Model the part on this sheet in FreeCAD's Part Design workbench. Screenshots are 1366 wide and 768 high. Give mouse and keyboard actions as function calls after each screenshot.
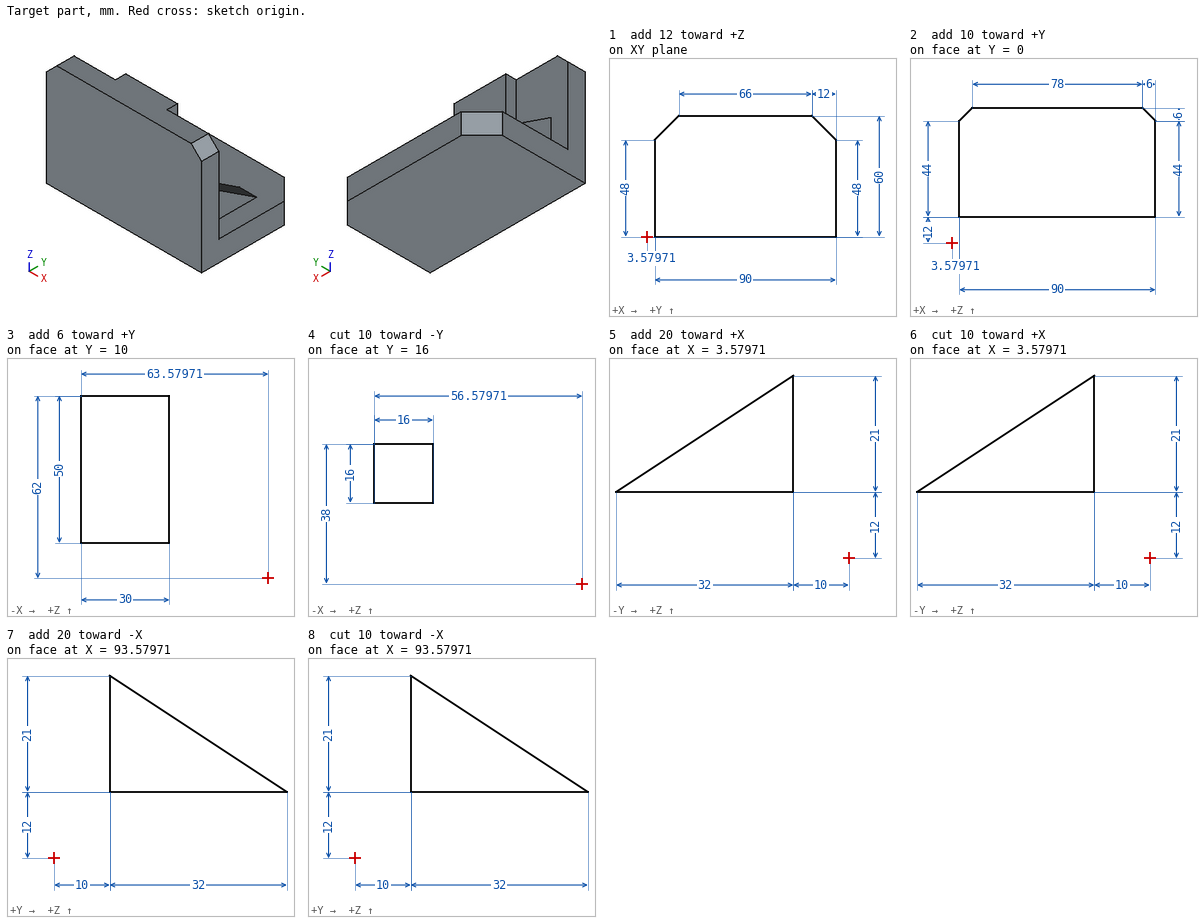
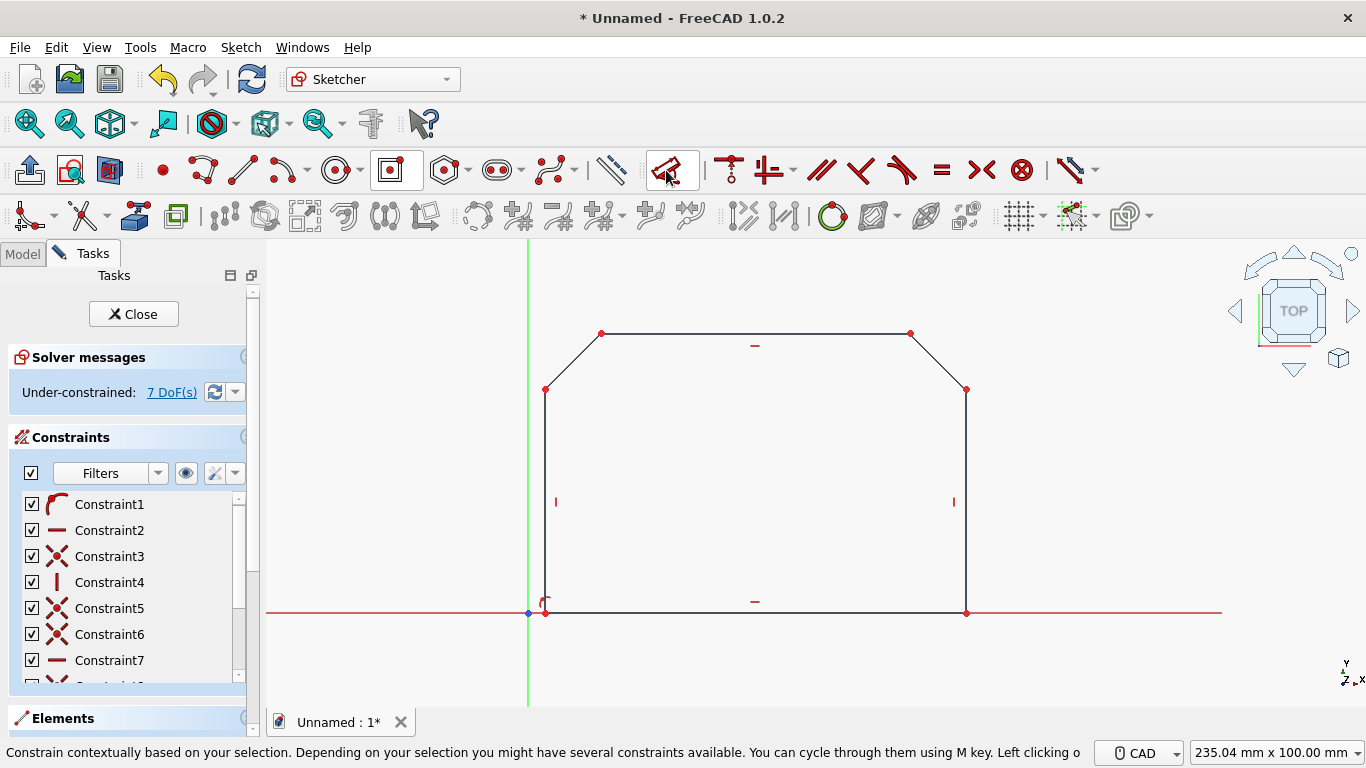
click(671, 613)
click(755, 647)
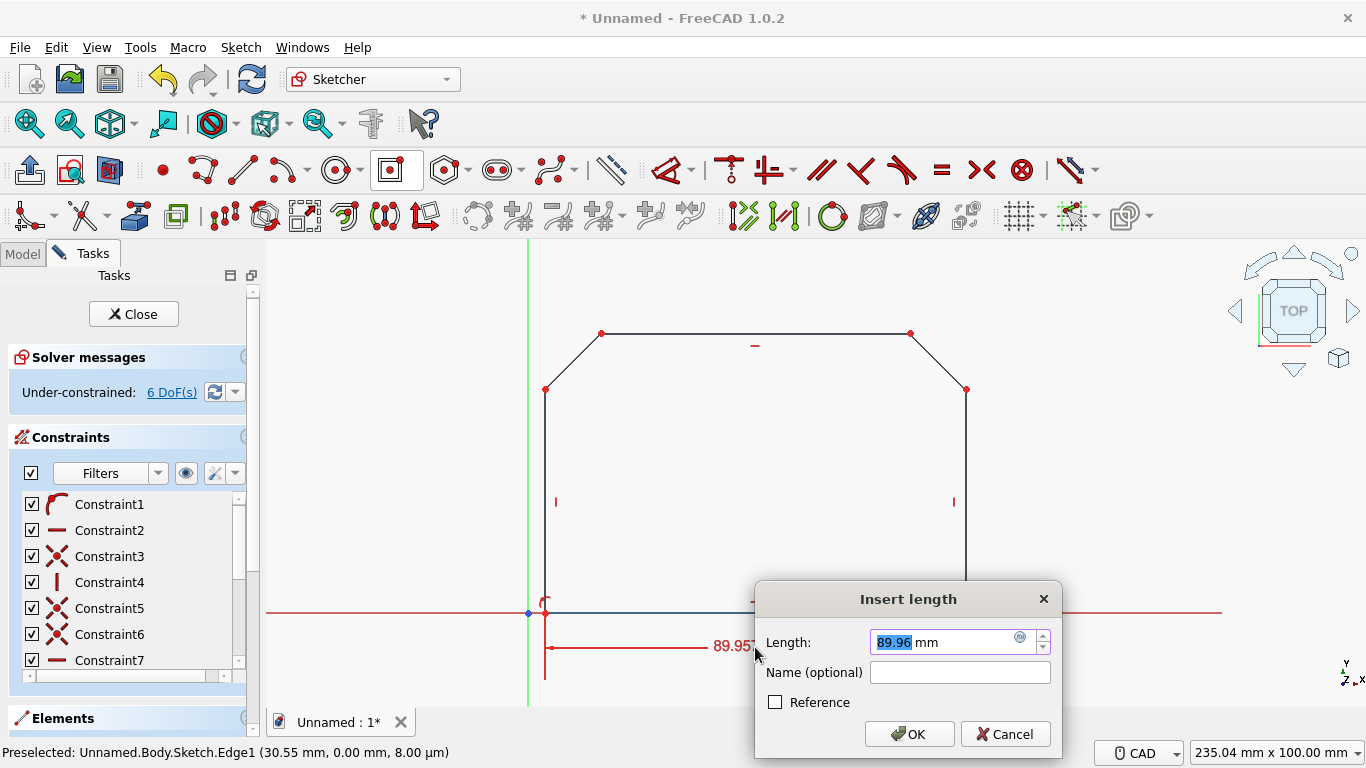
text(90)
key(Return)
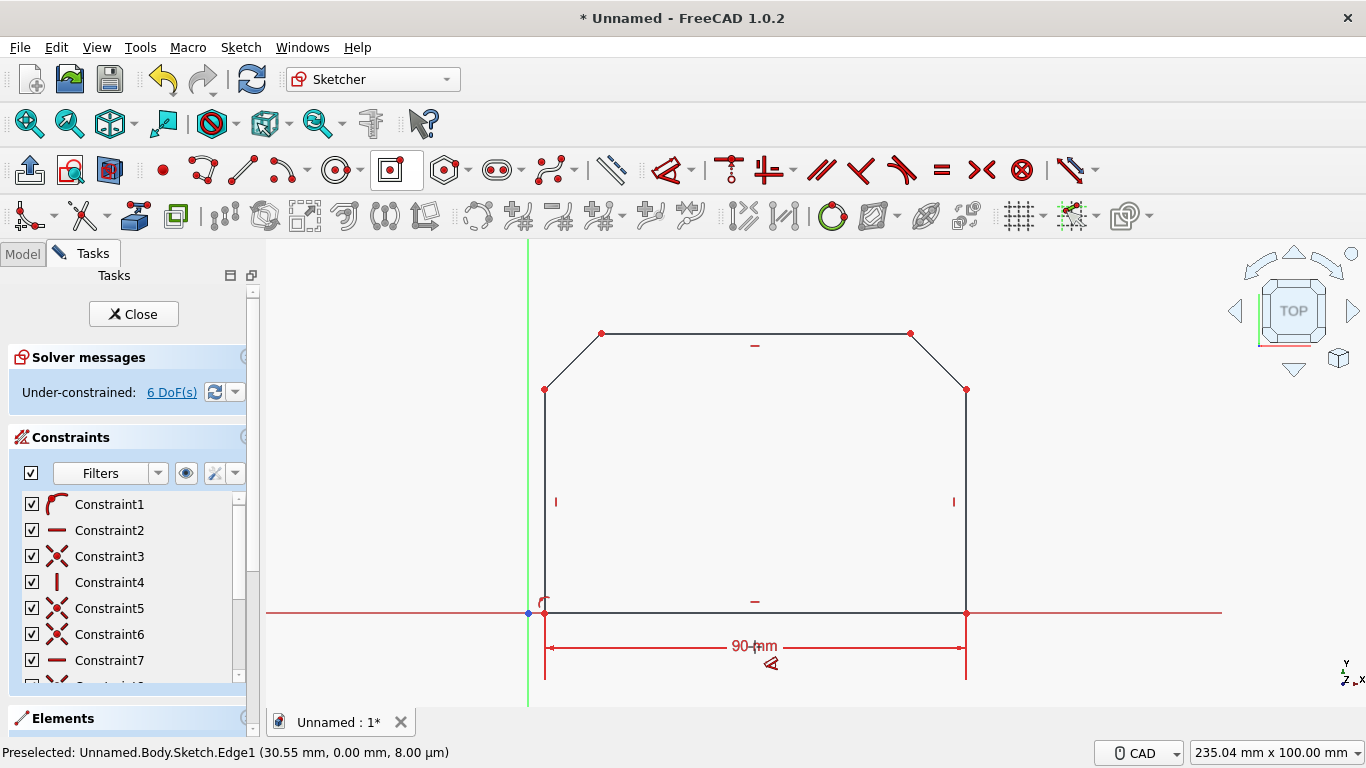
click(966, 546)
click(1000, 502)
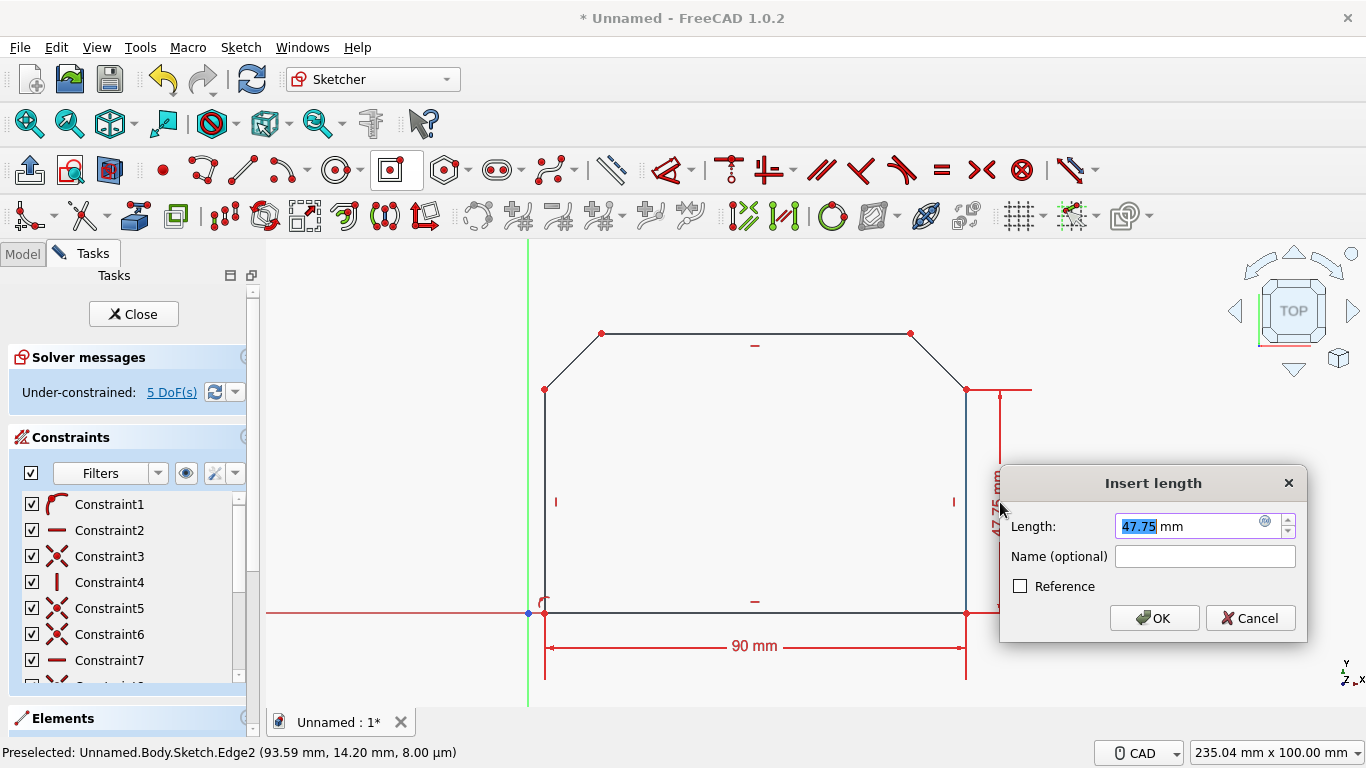
text(48)
key(Return)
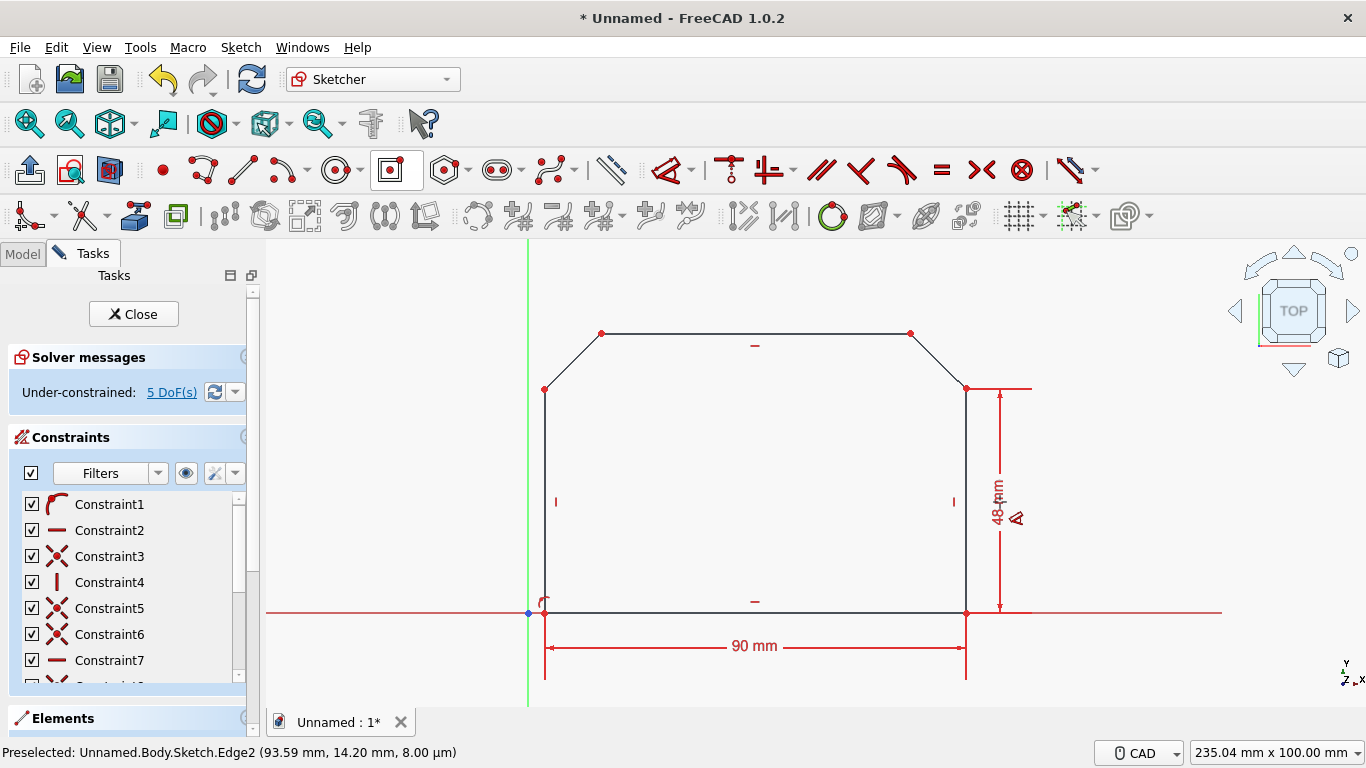
click(817, 334)
click(755, 300)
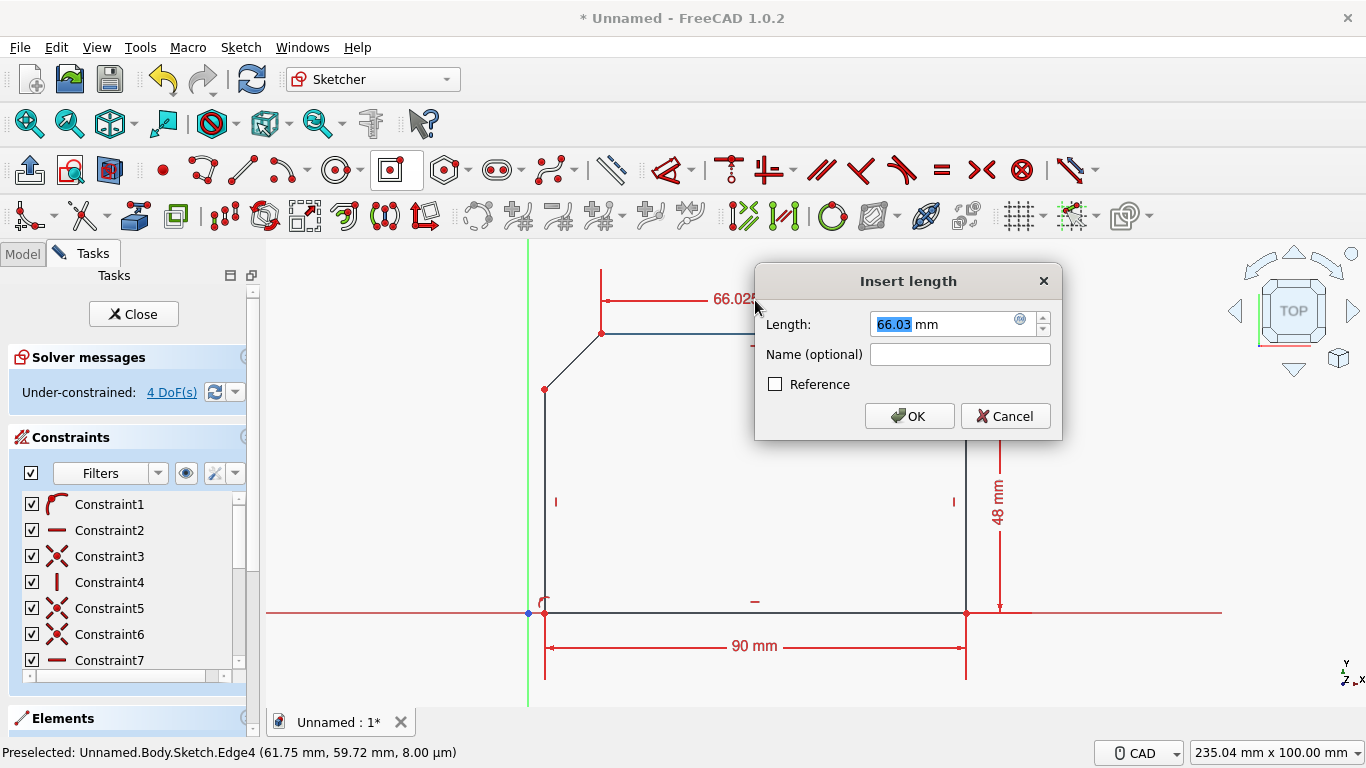
text(66)
key(Return)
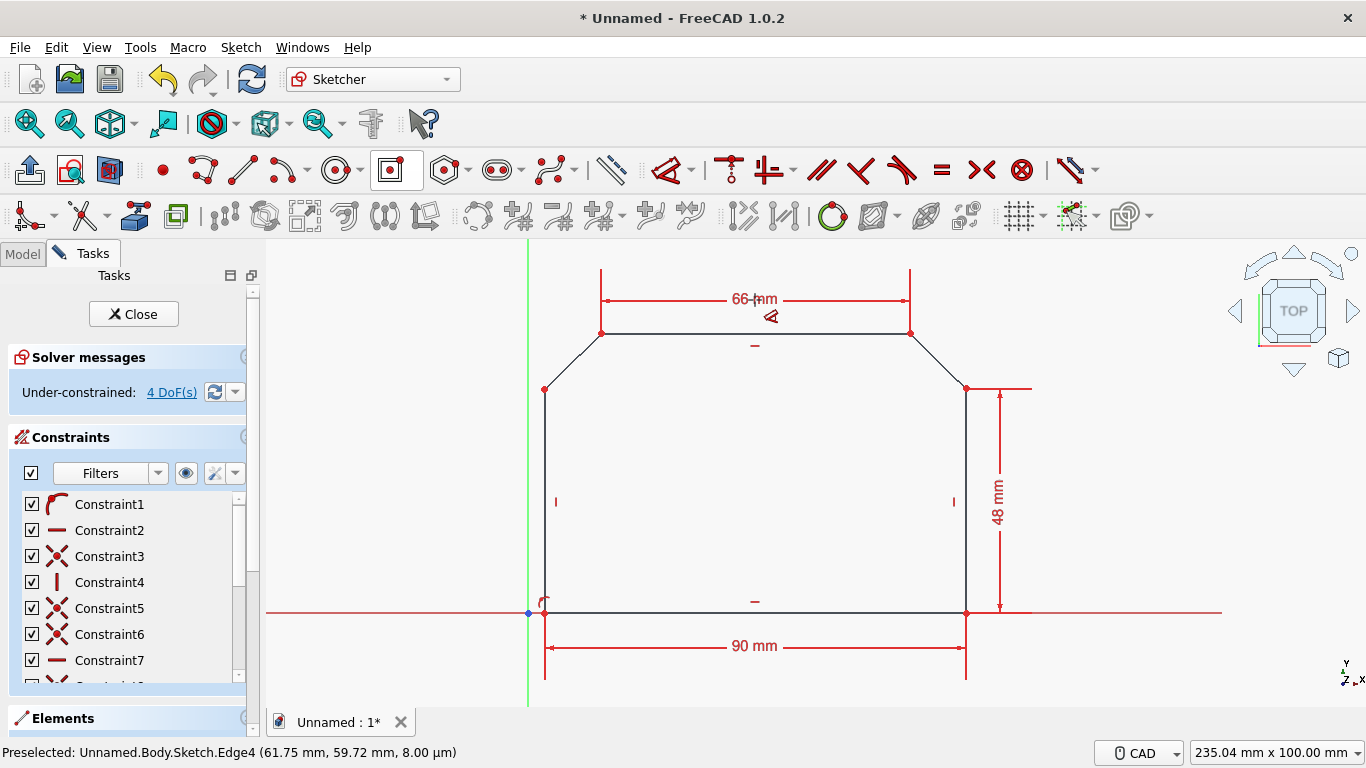
click(545, 457)
click(511, 502)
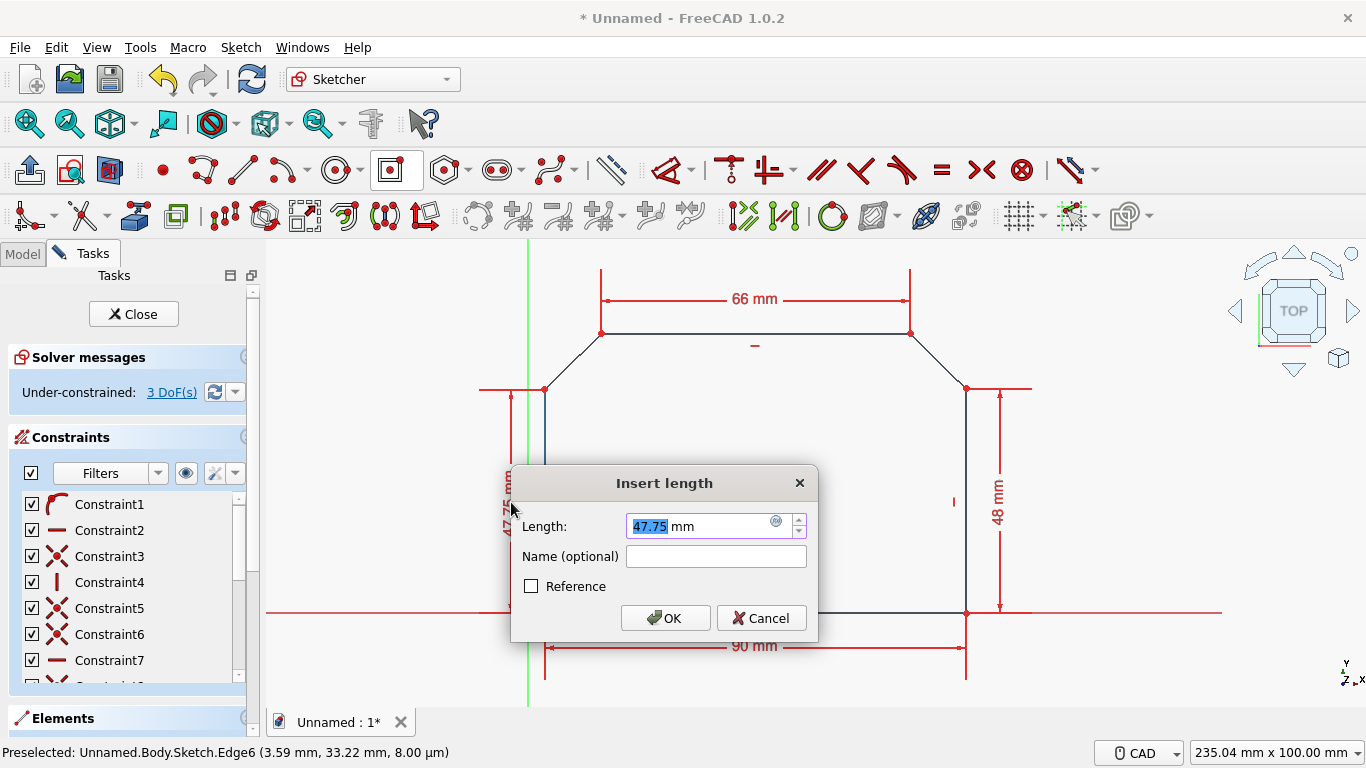
text(48)
key(Return)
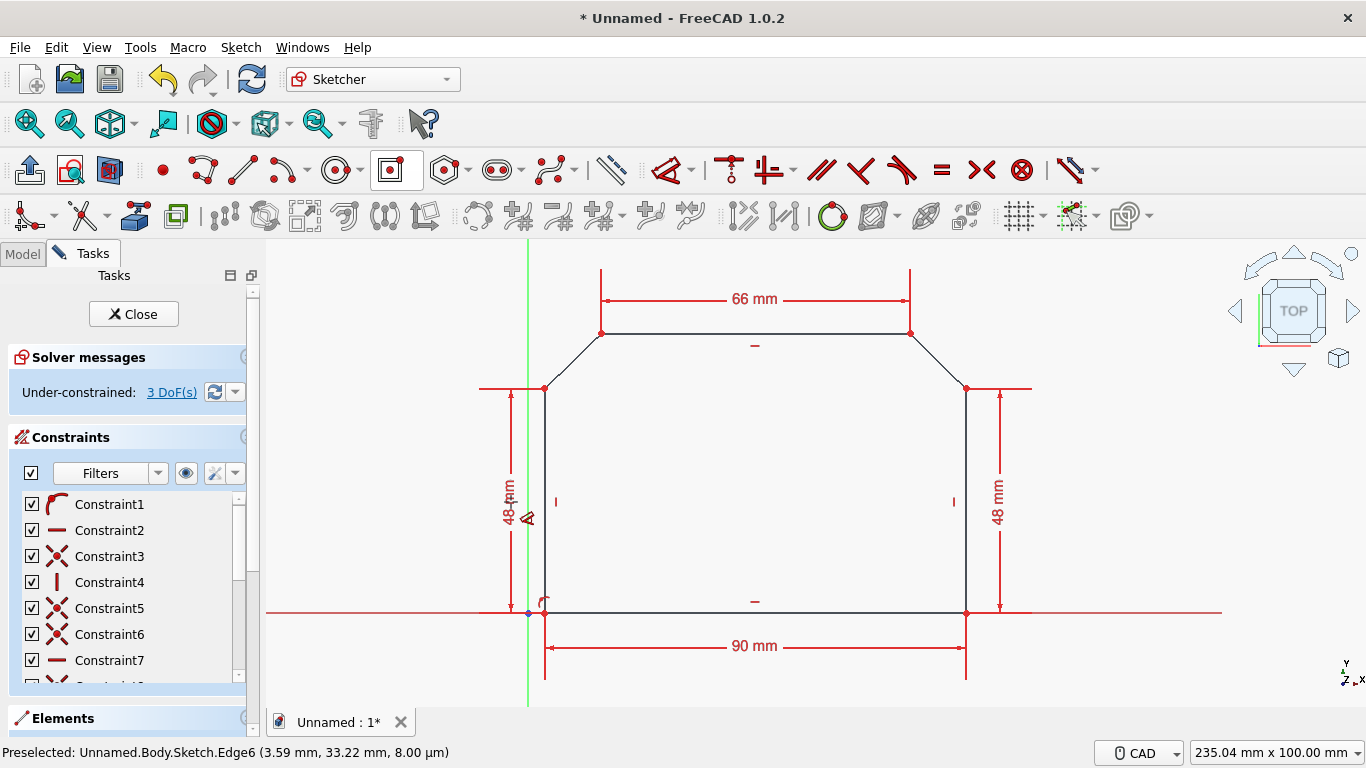
click(910, 334)
click(494, 474)